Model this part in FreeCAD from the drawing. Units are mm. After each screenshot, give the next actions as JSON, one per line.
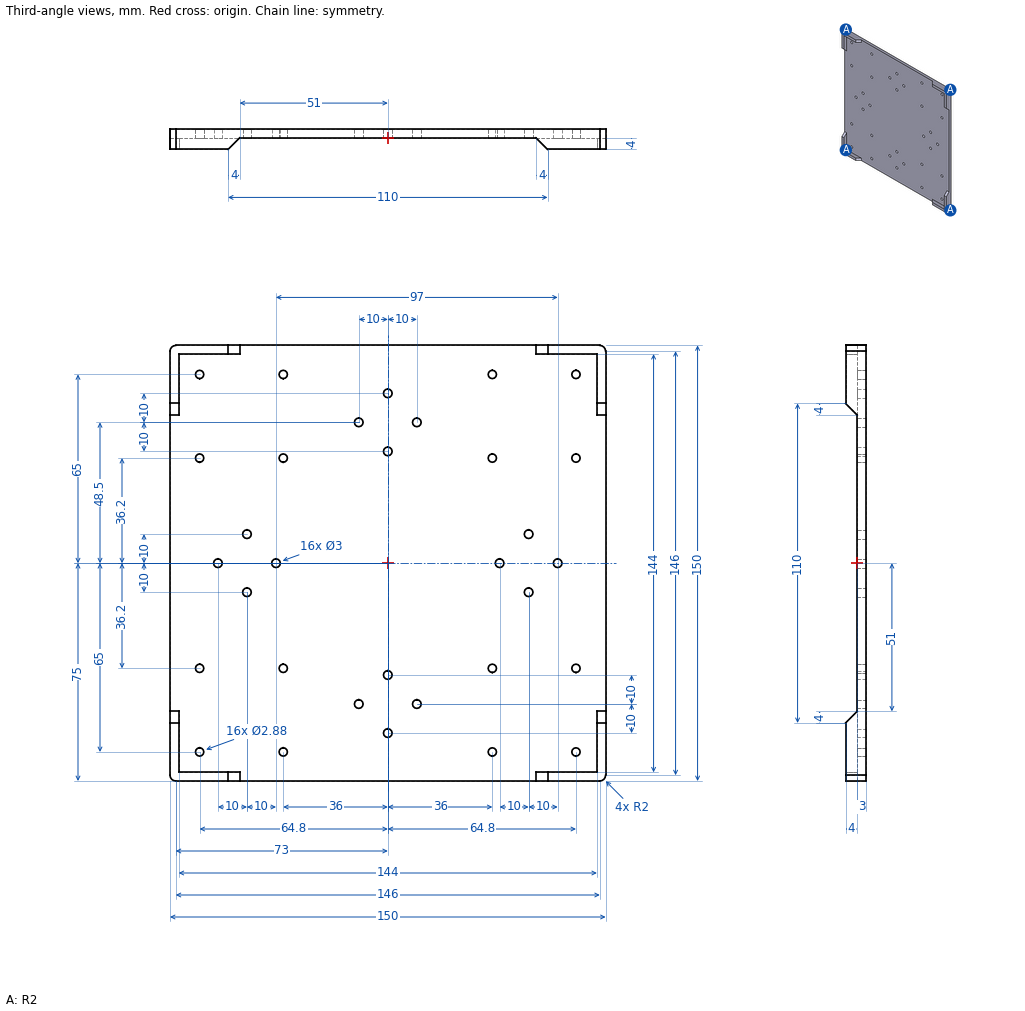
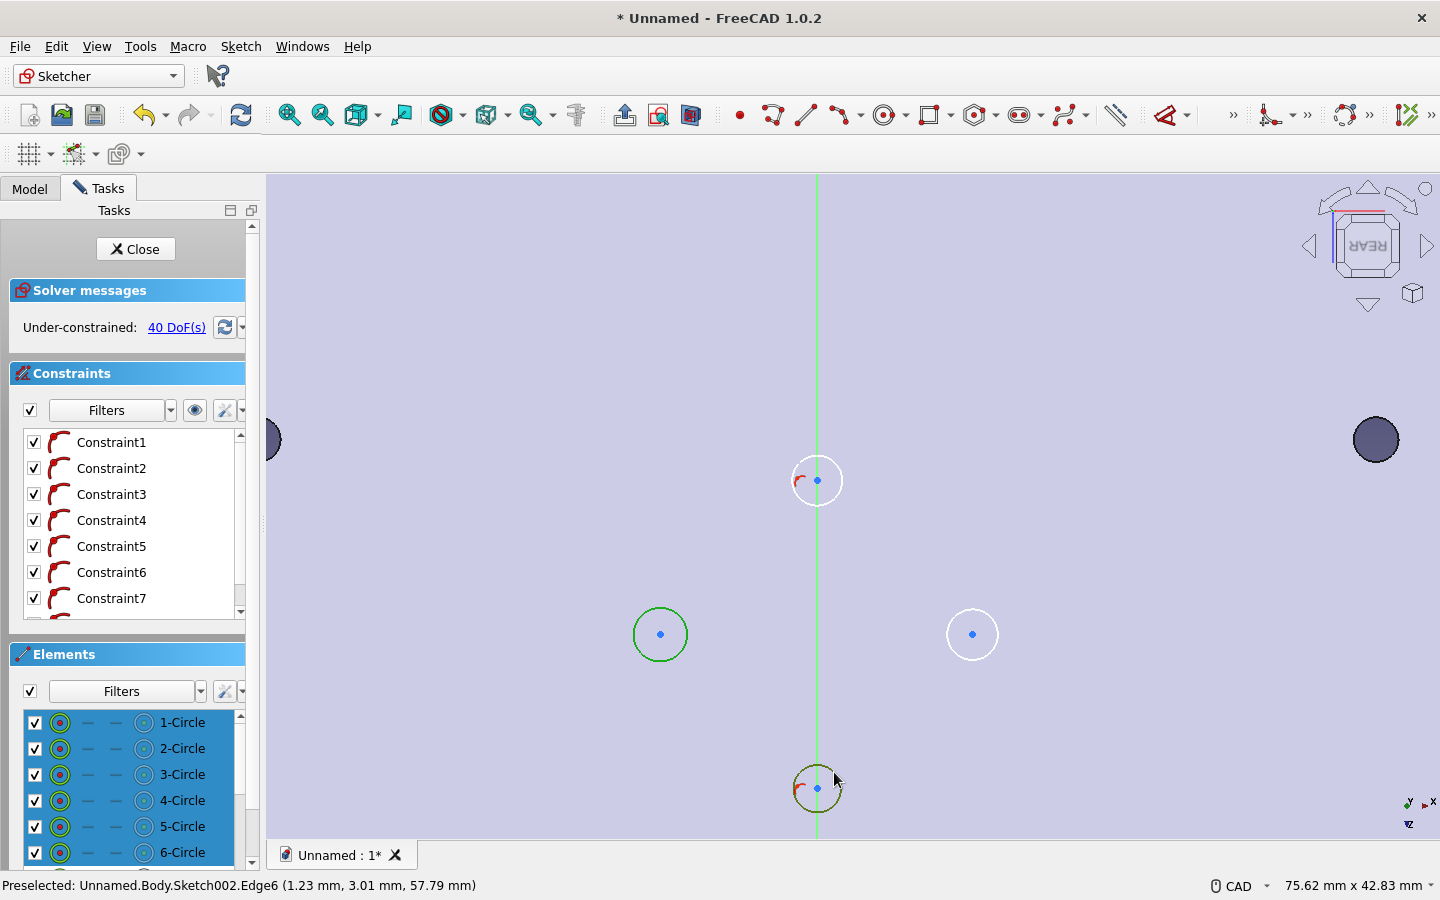
{"action": "left_click", "coordinate": [990, 617]}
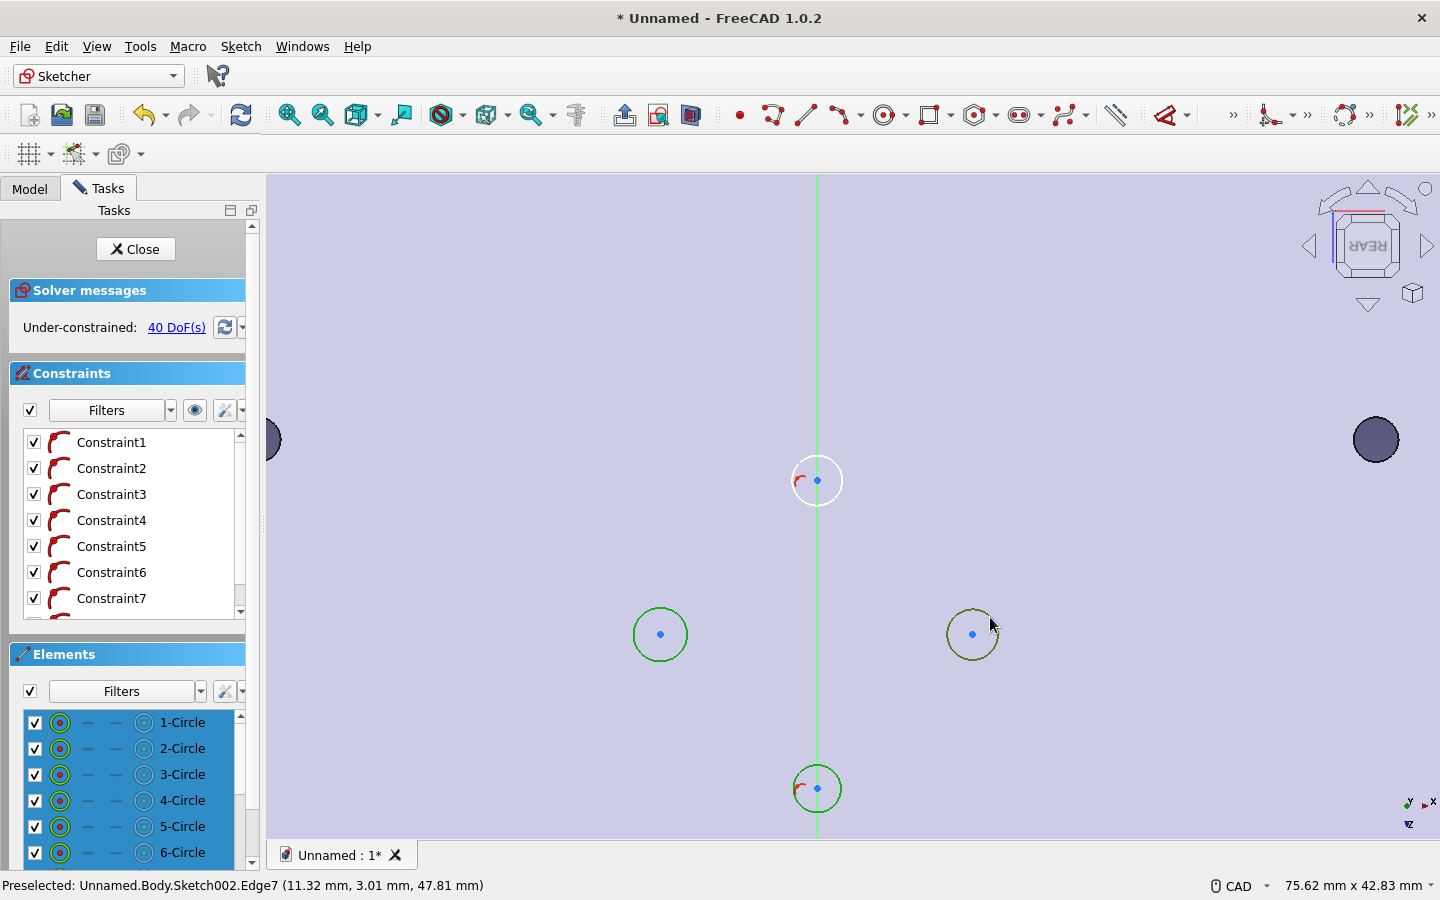
{"action": "left_click", "coordinate": [835, 463]}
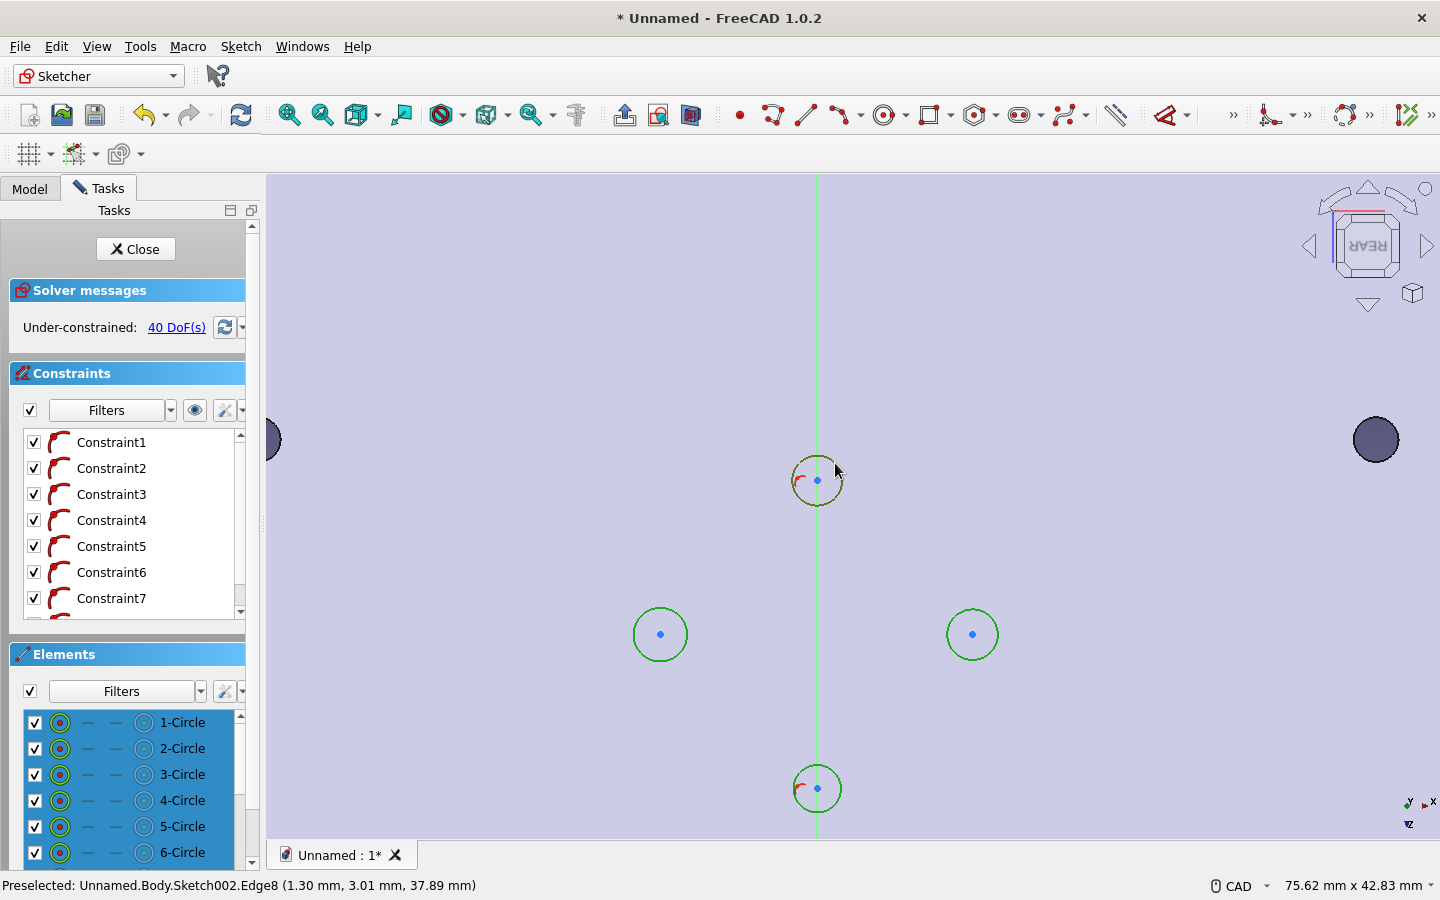
{"action": "scroll", "coordinate": [774, 712], "scroll_direction": "down", "scroll_amount": 7}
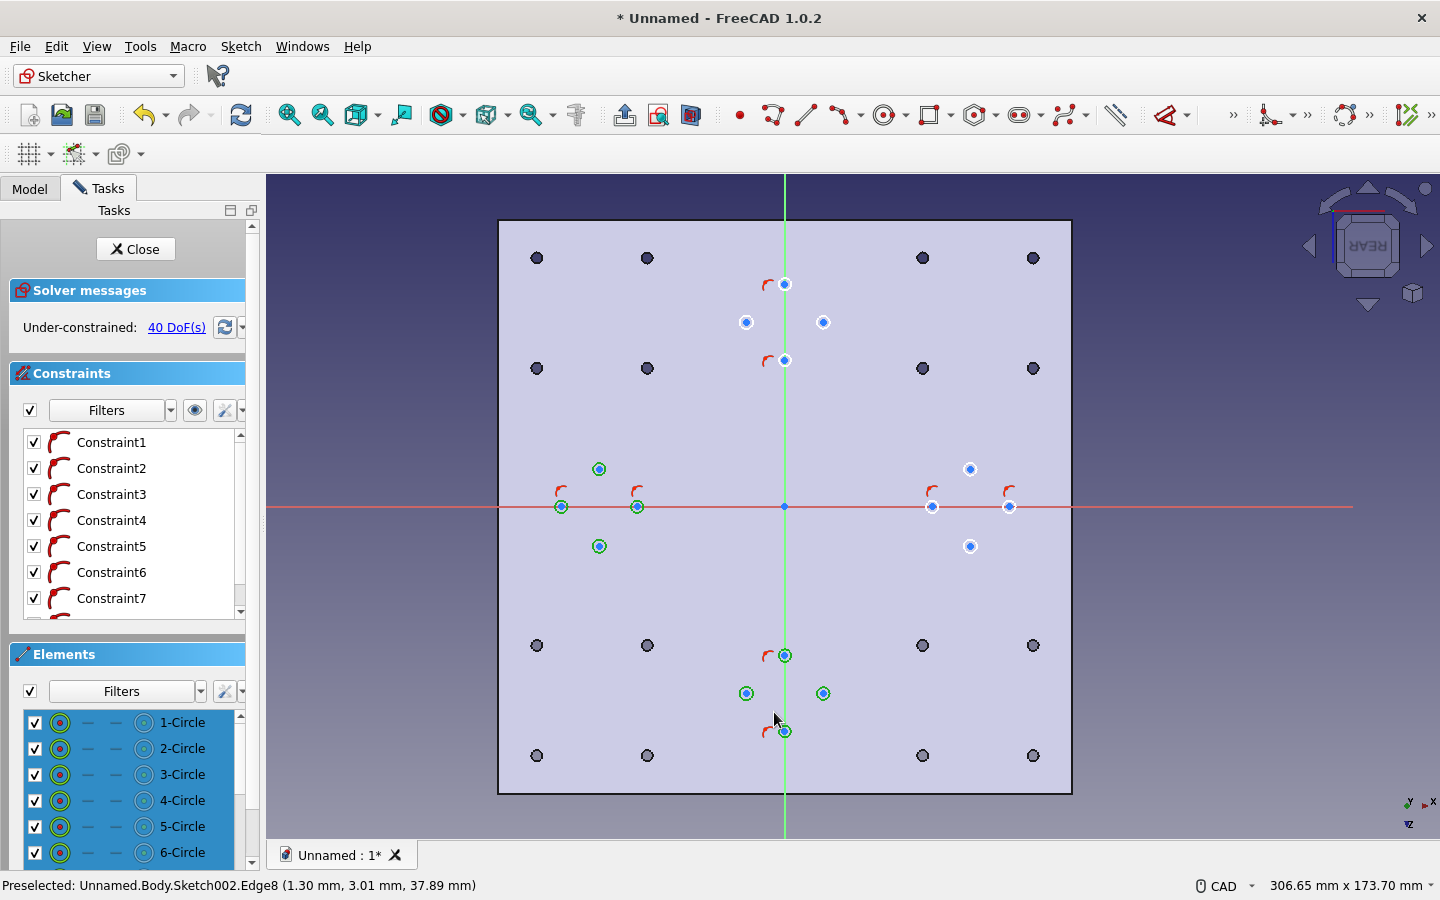
{"action": "scroll", "coordinate": [1014, 502], "scroll_direction": "up", "scroll_amount": 6}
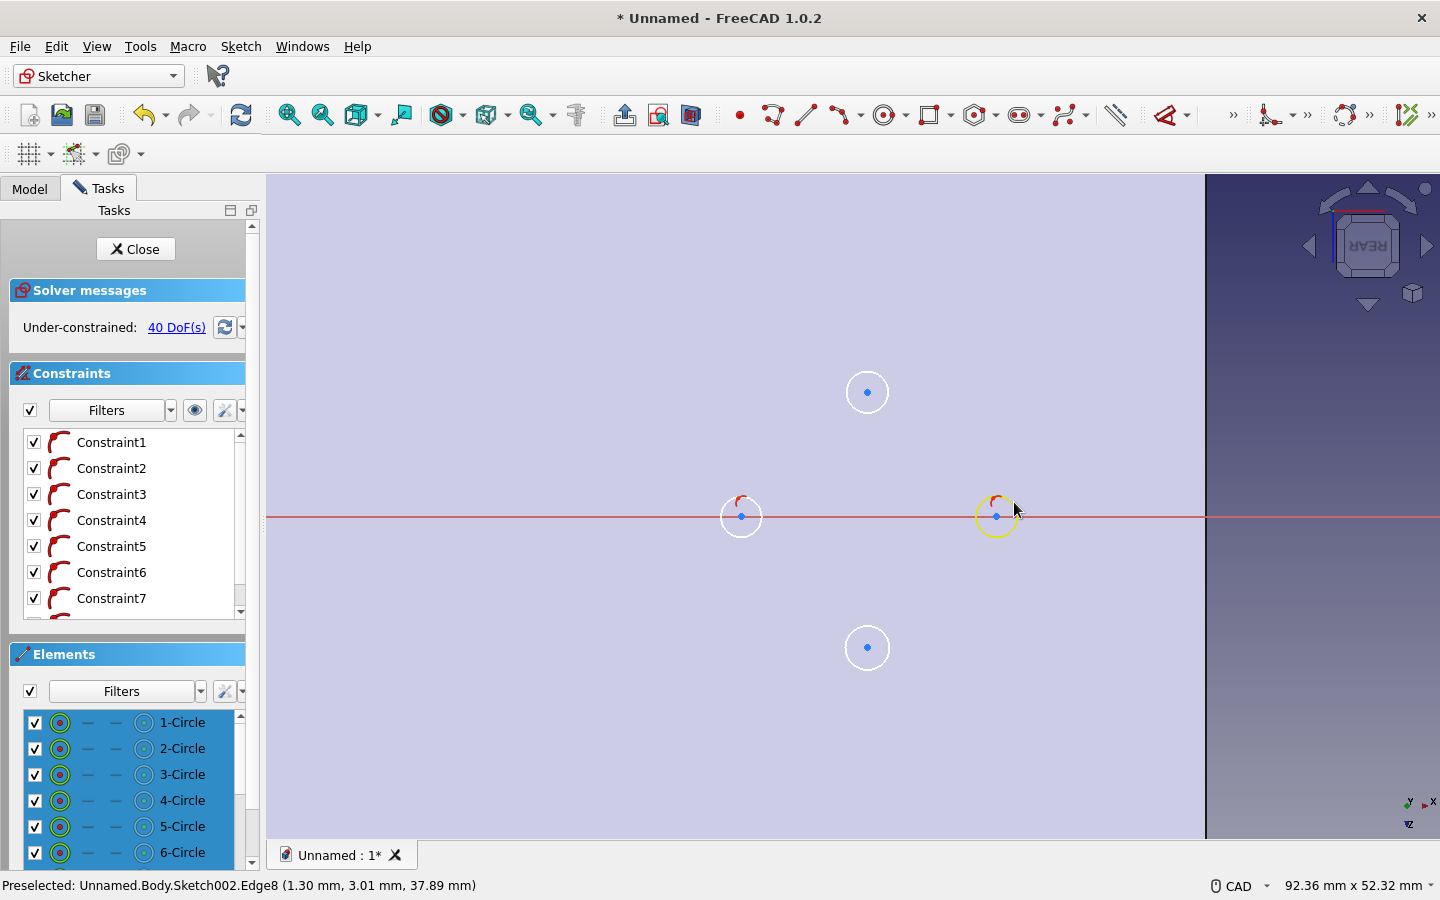
{"action": "left_click", "coordinate": [1011, 502]}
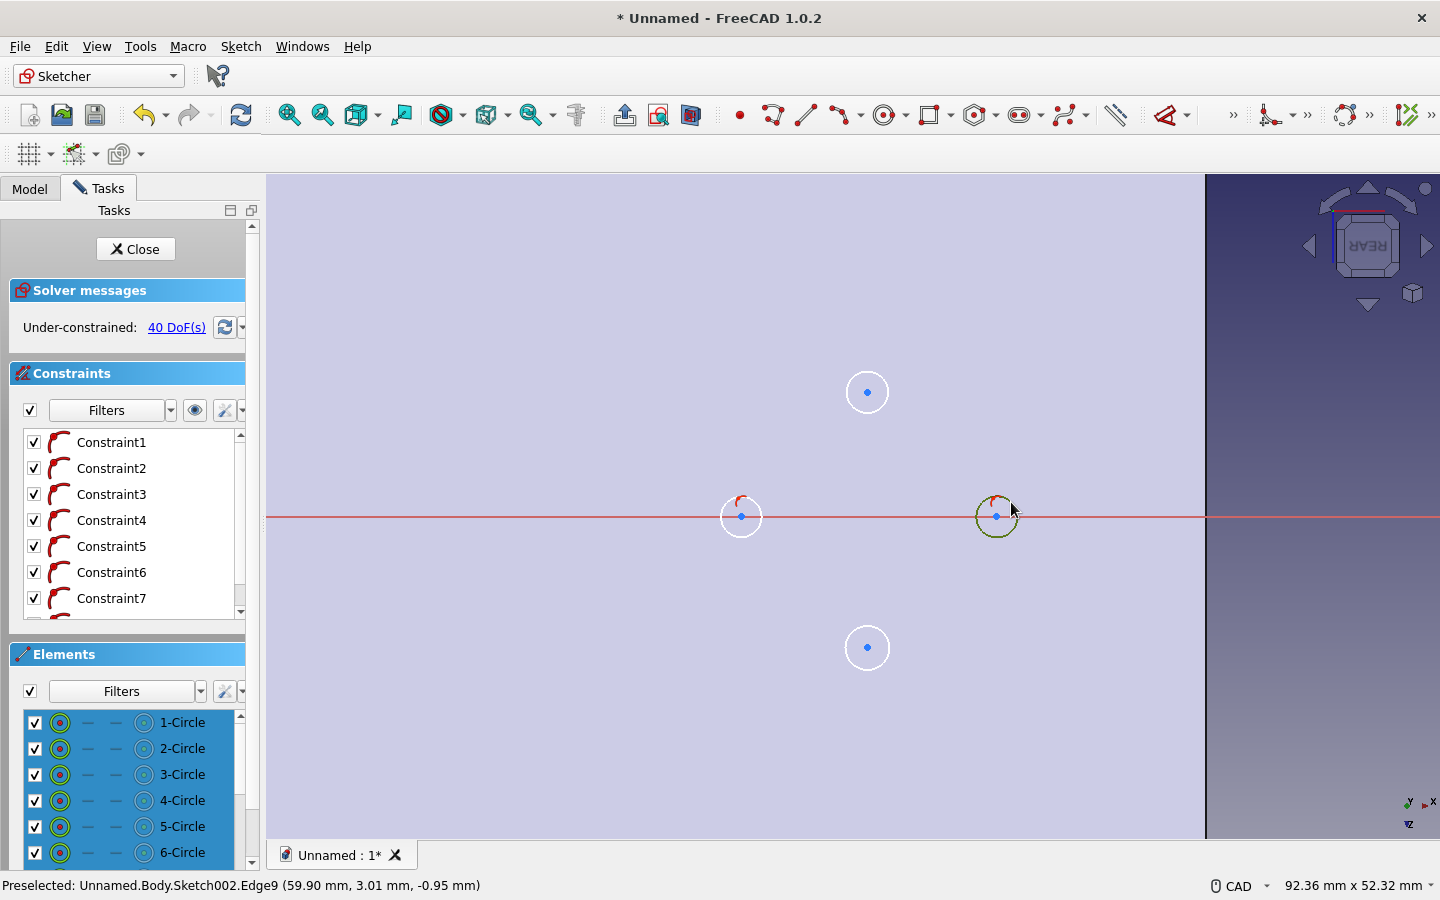
{"action": "left_click", "coordinate": [882, 378]}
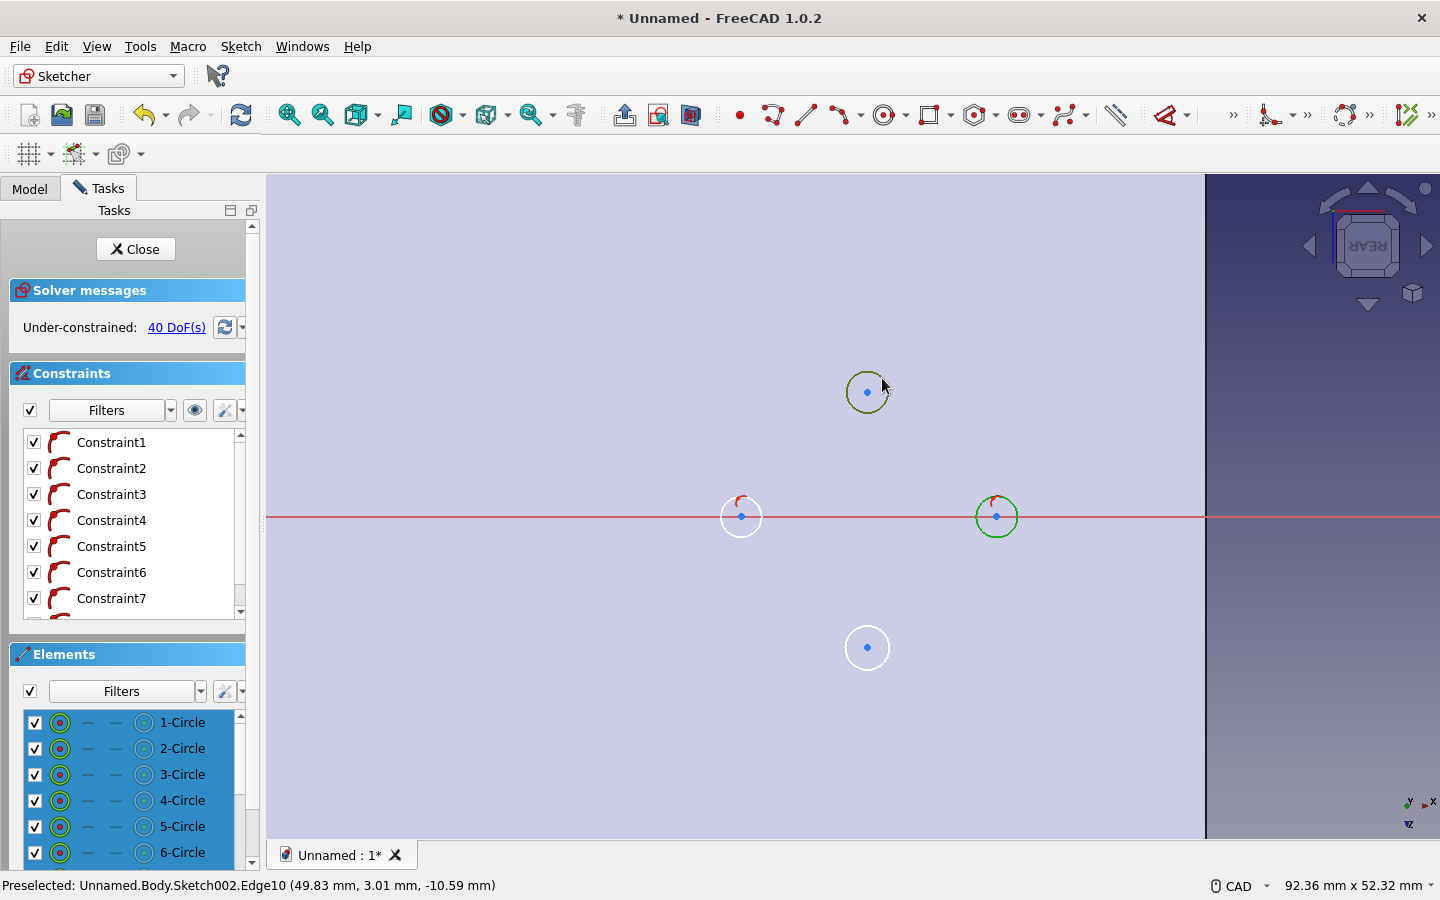
{"action": "left_click", "coordinate": [756, 503]}